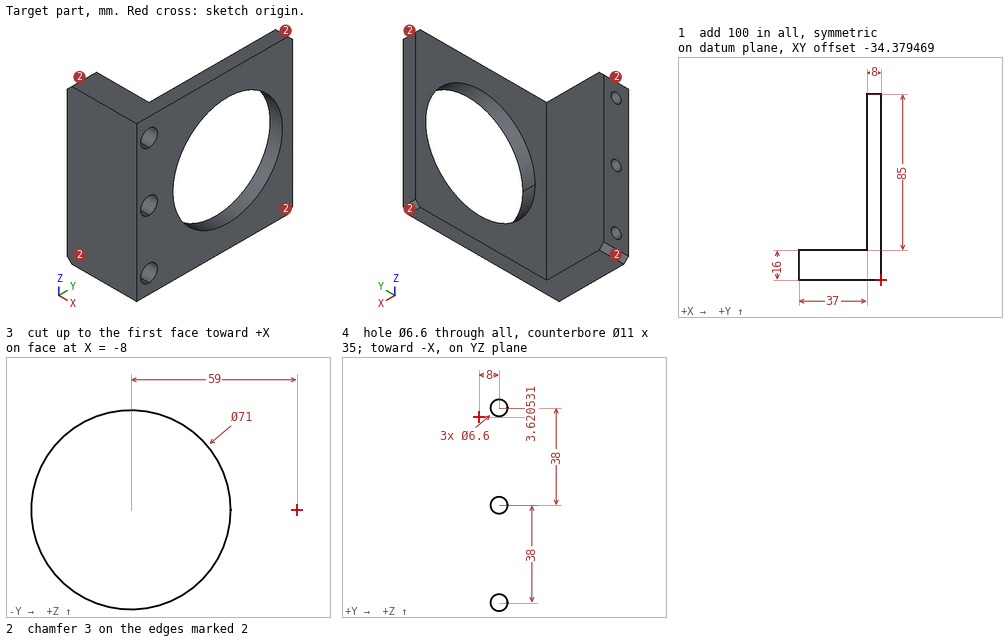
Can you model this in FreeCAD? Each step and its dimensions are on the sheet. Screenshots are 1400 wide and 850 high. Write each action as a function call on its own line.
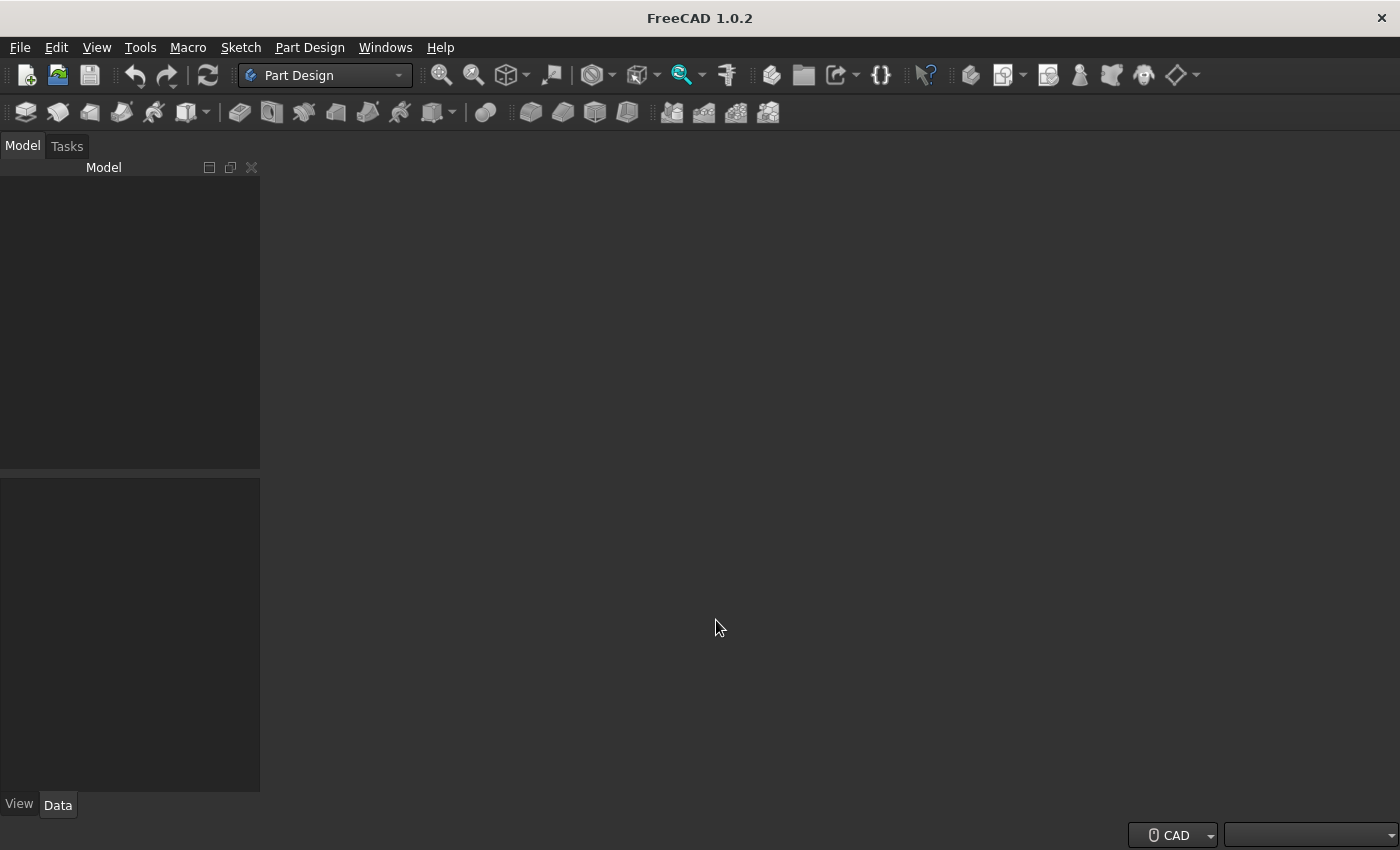
click(26, 76)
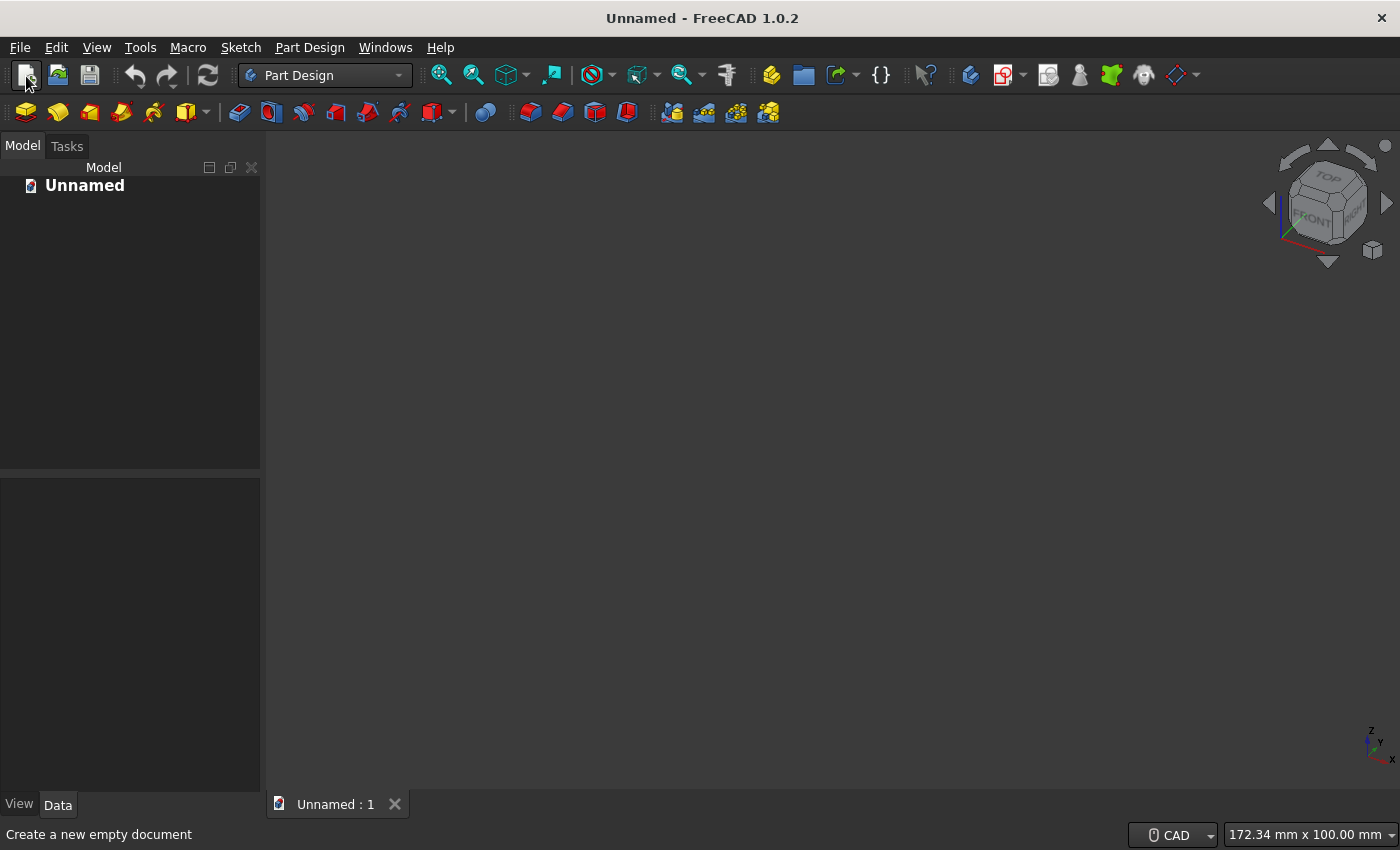
click(972, 76)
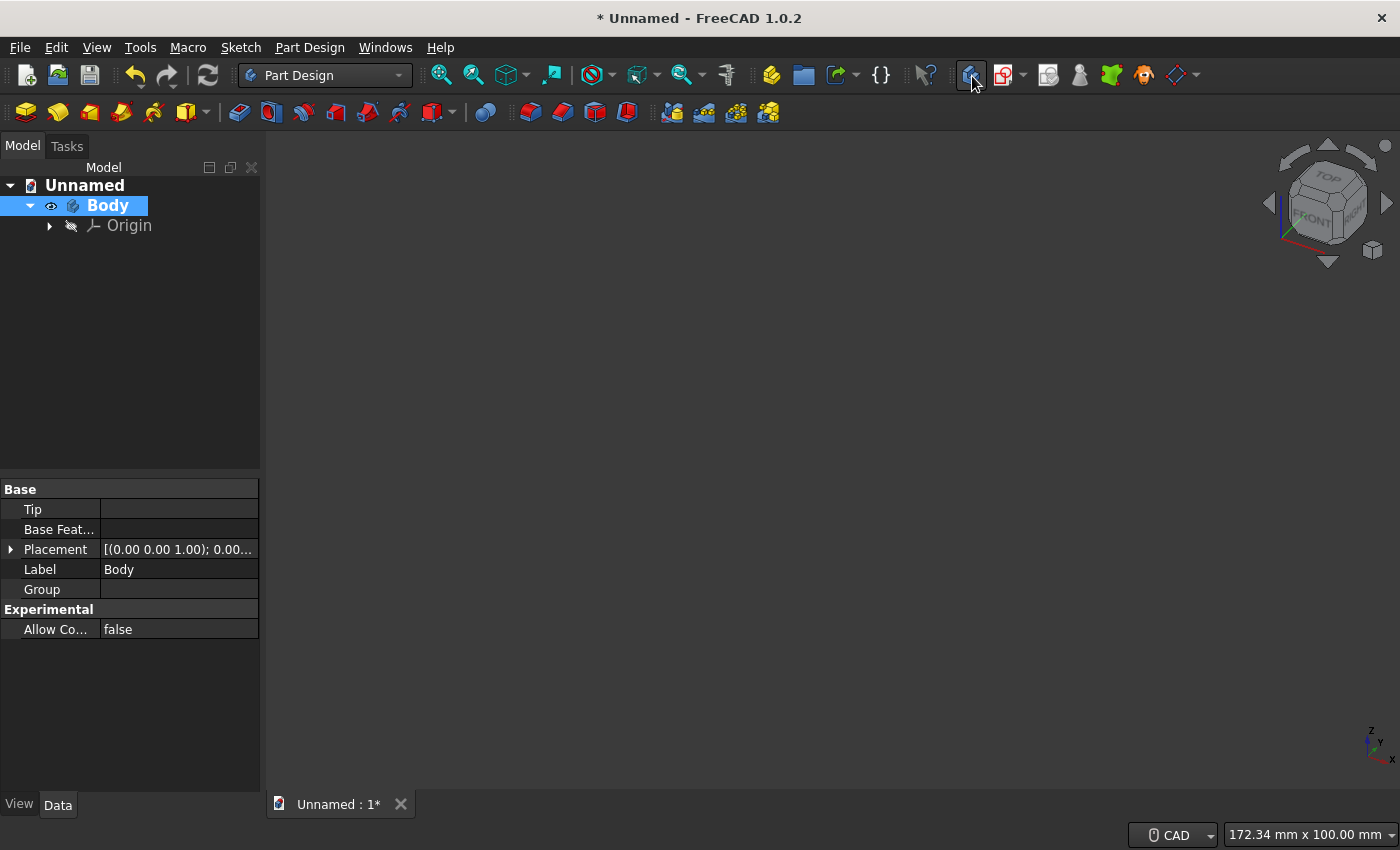
click(50, 226)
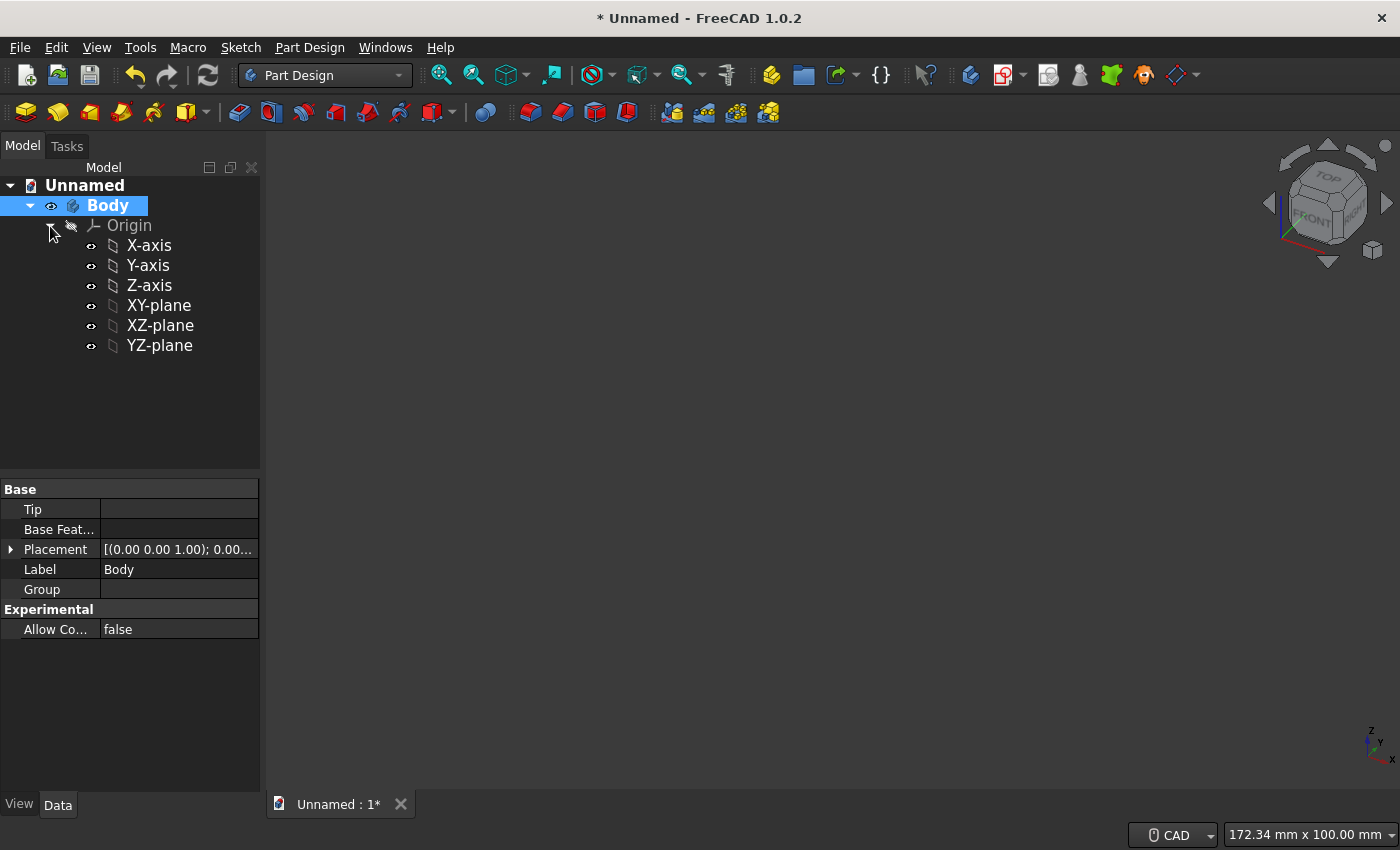
click(136, 306)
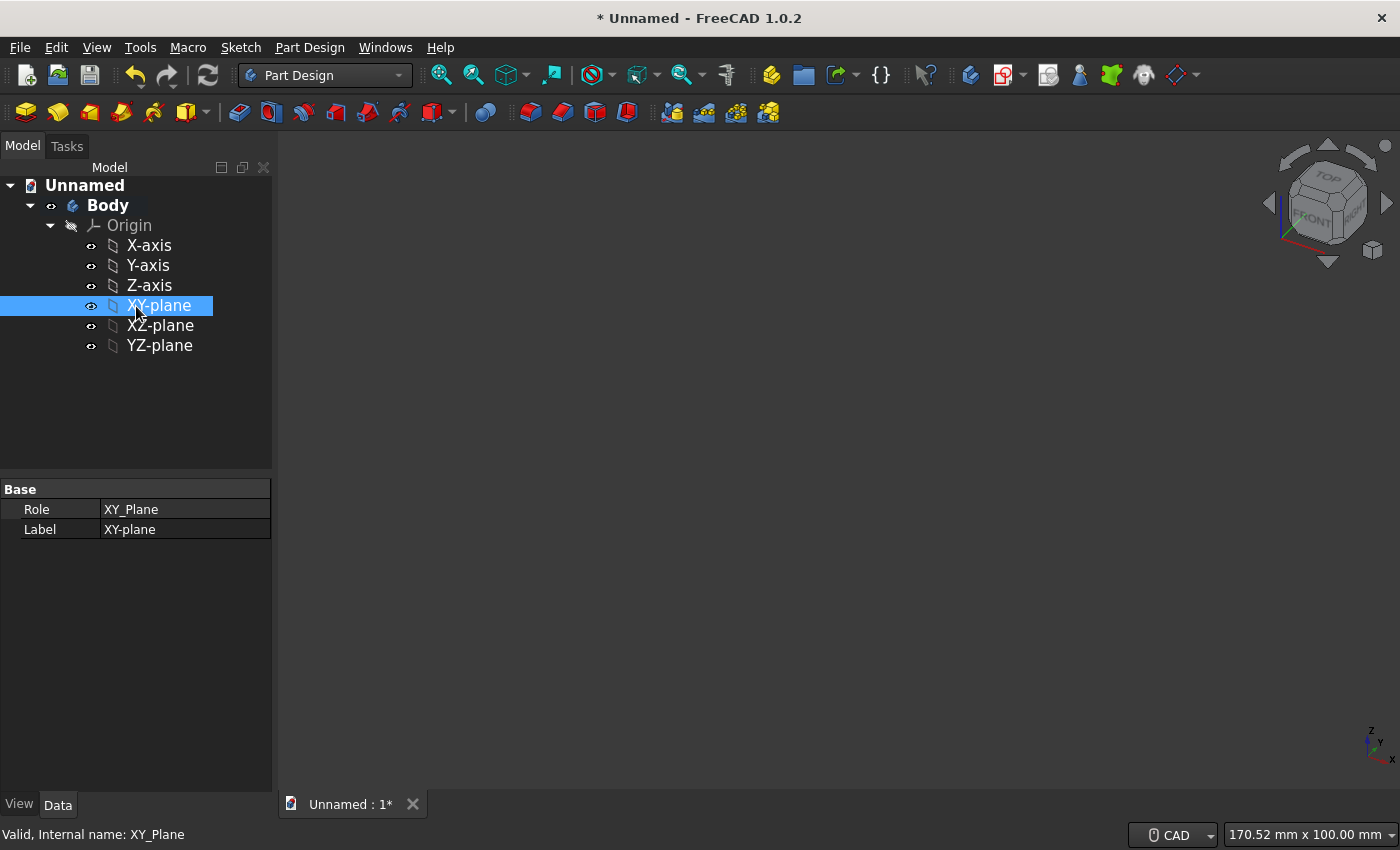
click(1176, 76)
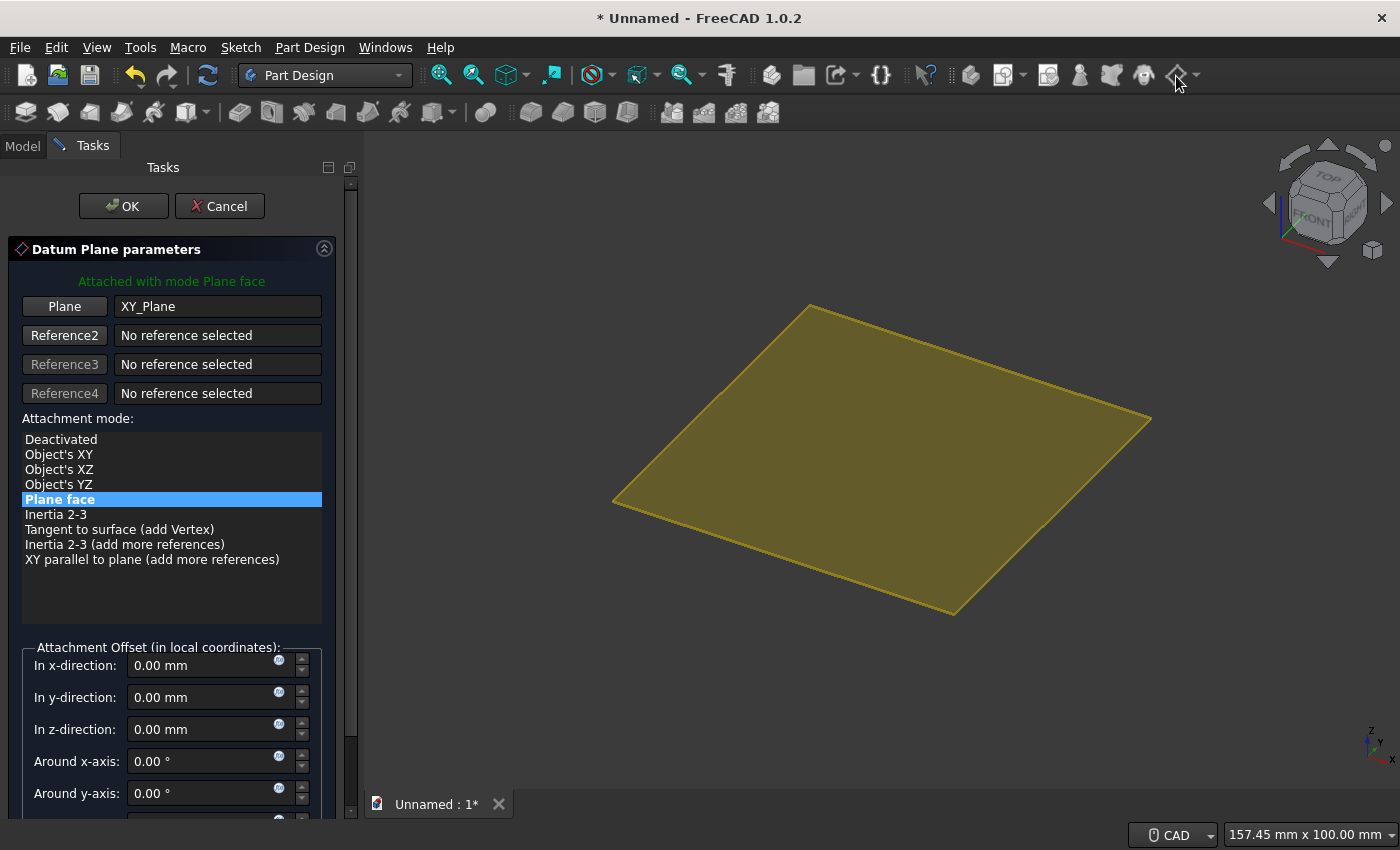
triple_click(210, 729)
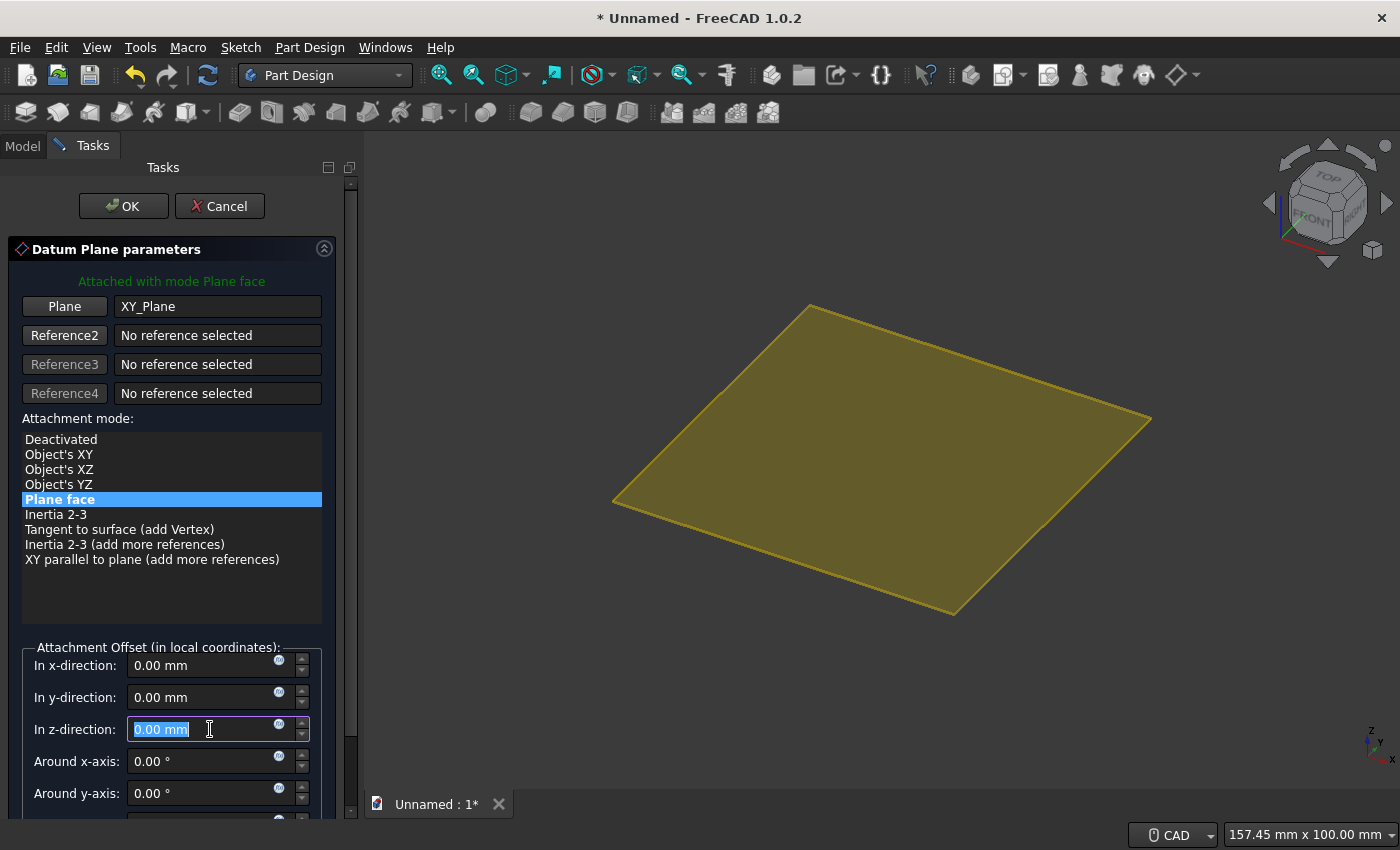
text(-34.379469)
key(Tab)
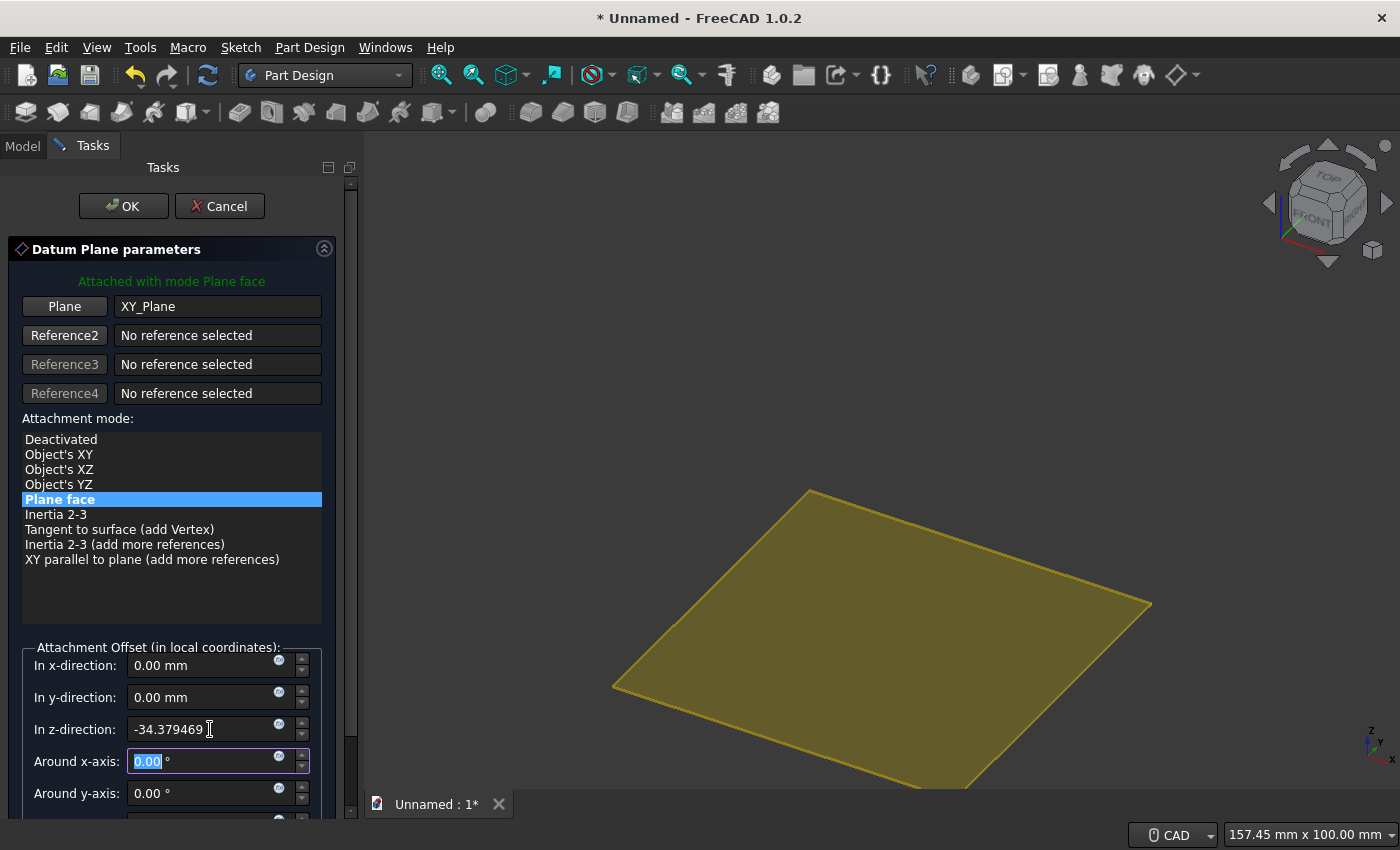
click(124, 206)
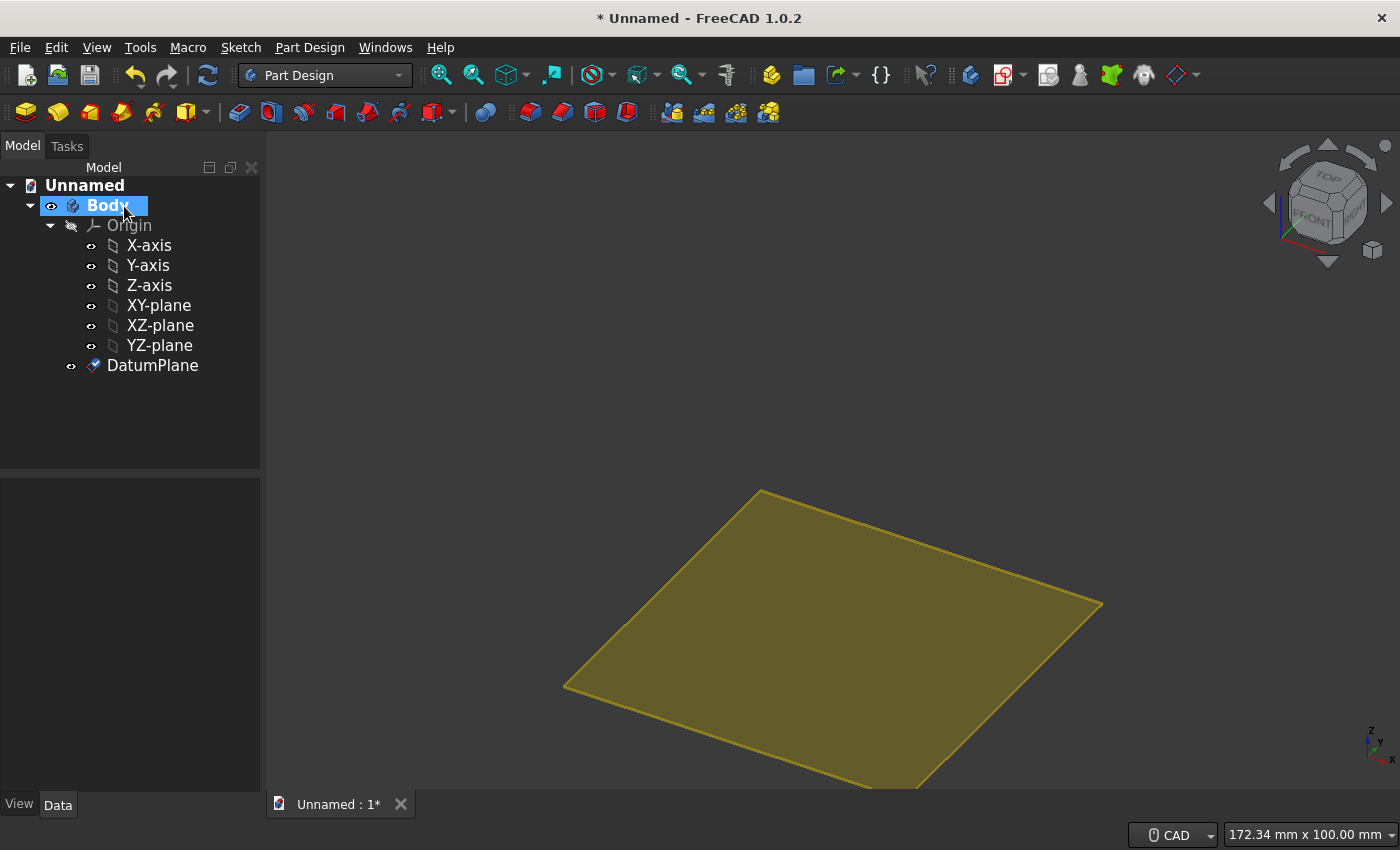
click(116, 366)